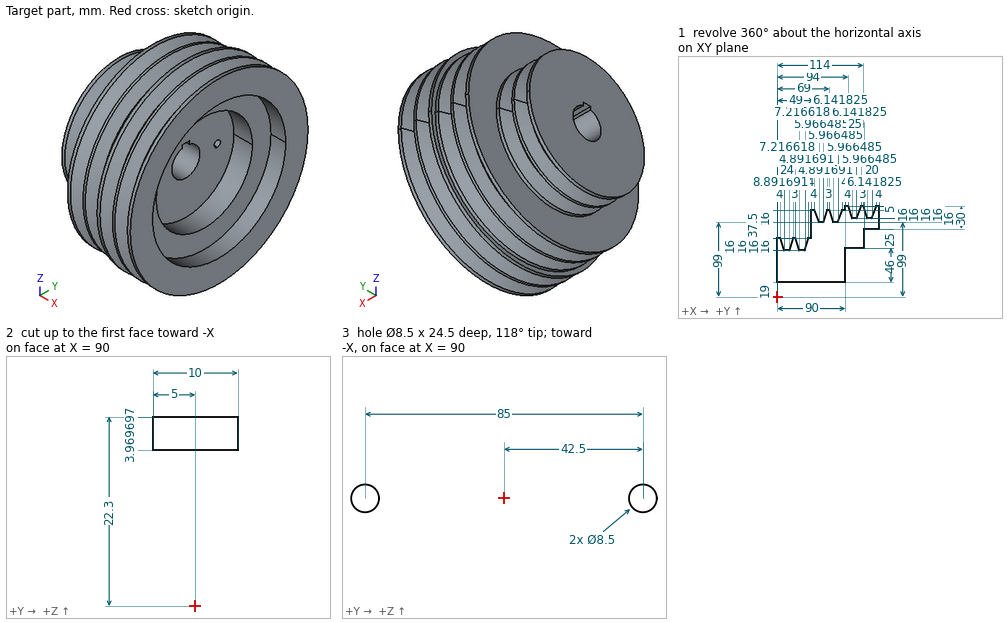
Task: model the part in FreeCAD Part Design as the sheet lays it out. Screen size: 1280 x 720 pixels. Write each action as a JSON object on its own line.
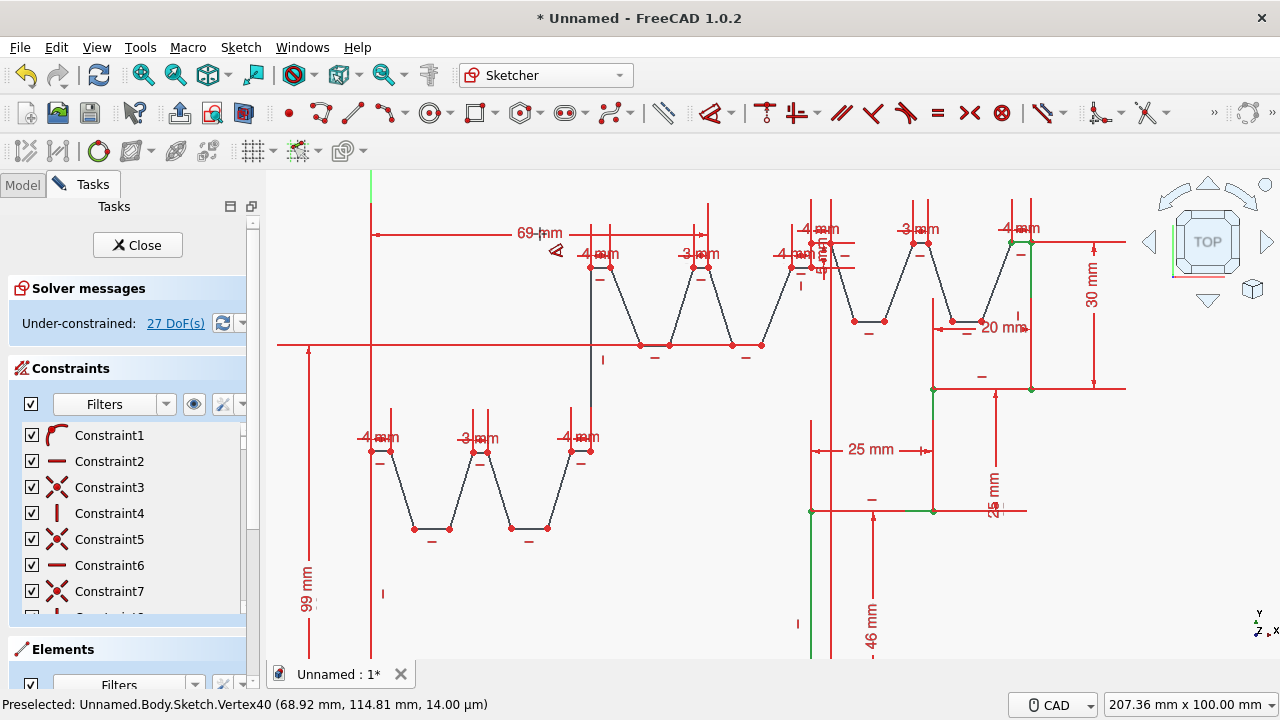
{"action": "left_click", "coordinate": [670, 346]}
{"action": "left_click", "coordinate": [337, 488]}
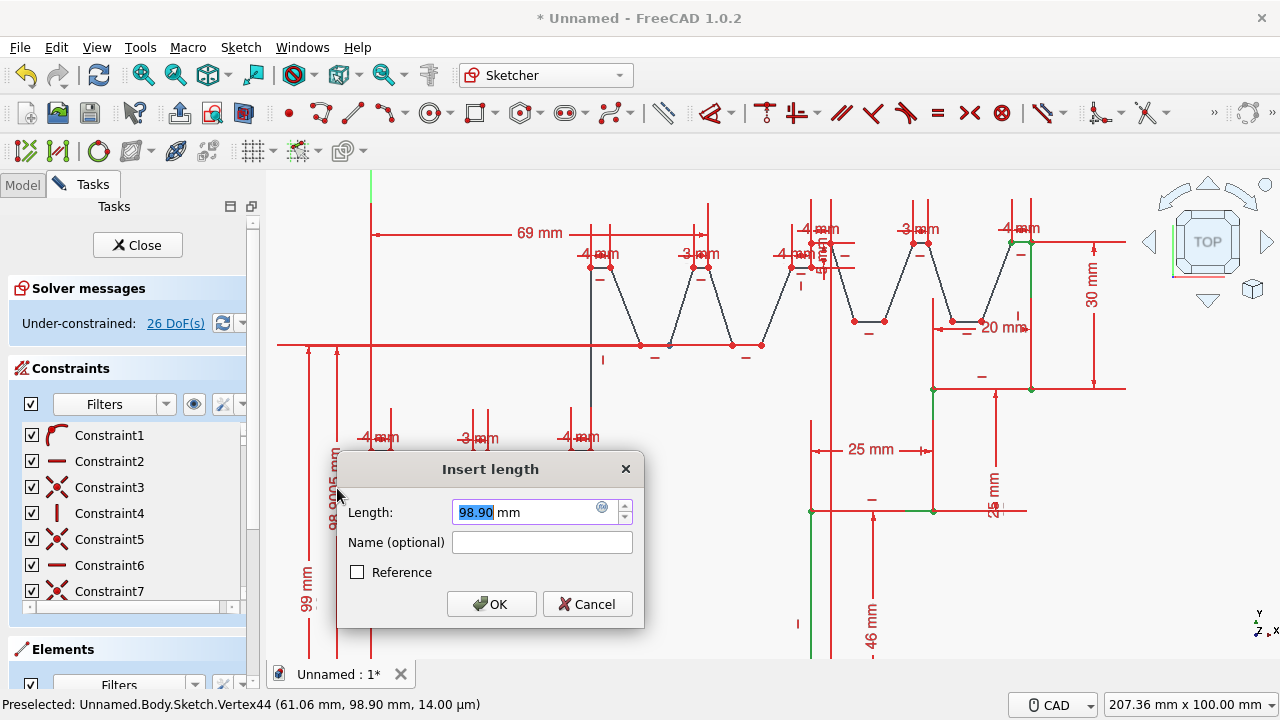
{"action": "type", "text": "99"}
{"action": "key", "text": "Return"}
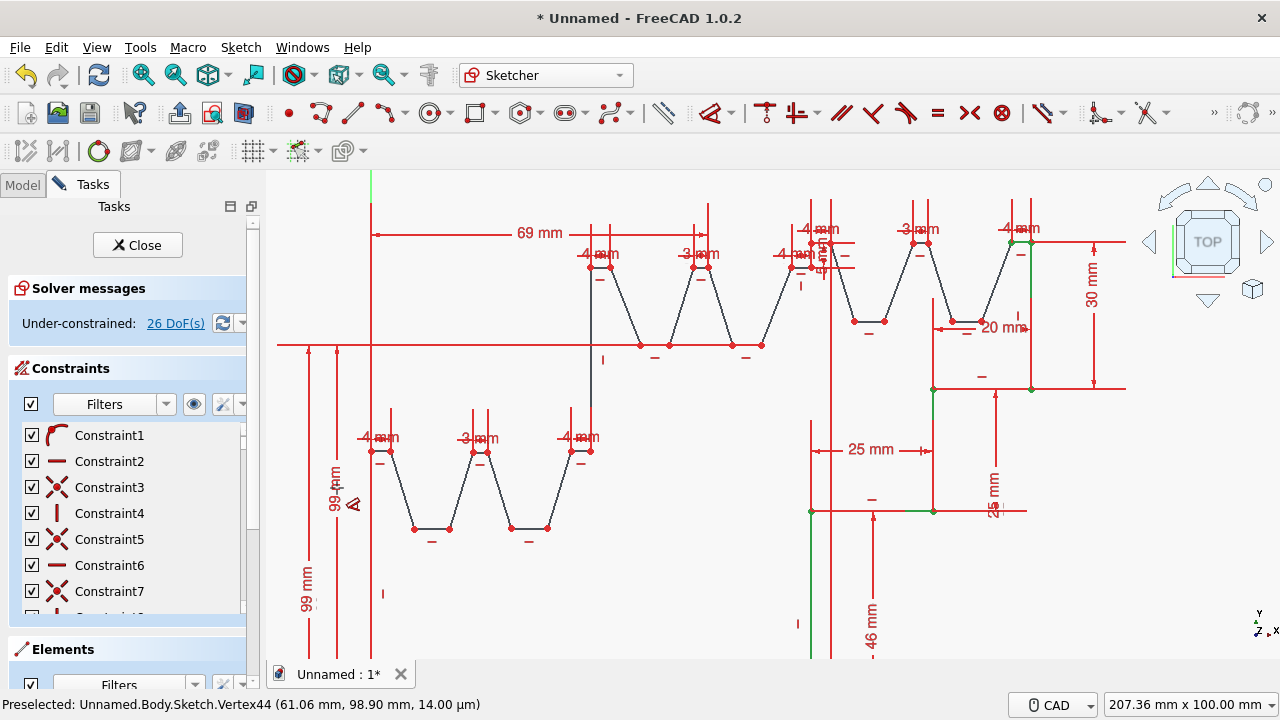
{"action": "left_click", "coordinate": [610, 268]}
{"action": "left_click", "coordinate": [436, 234]}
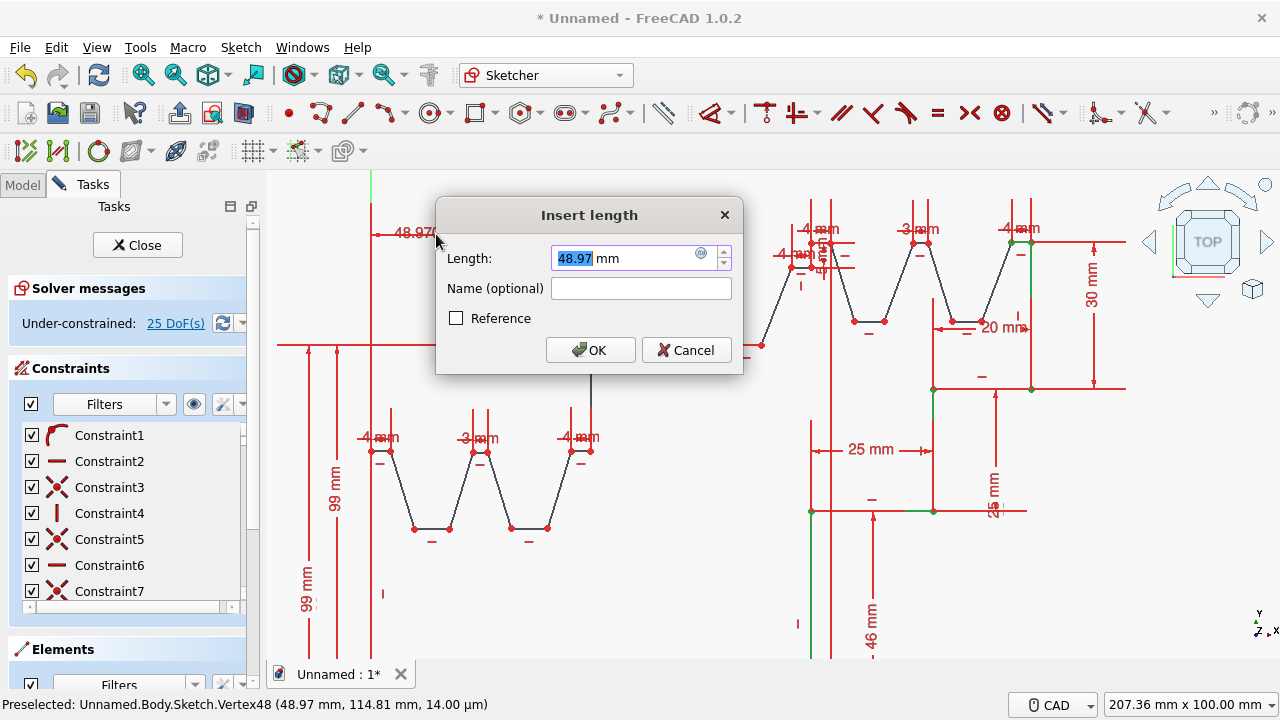
{"action": "type", "text": "49"}
{"action": "key", "text": "Return"}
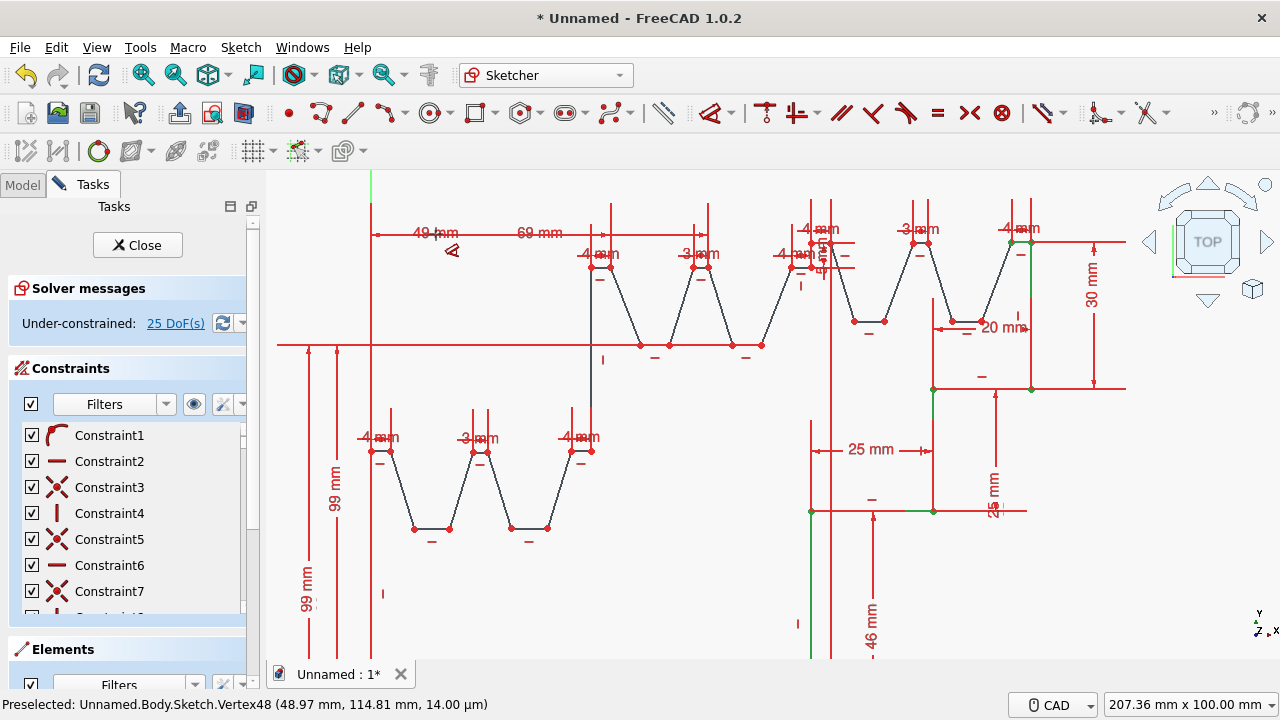
{"action": "left_click", "coordinate": [488, 453]}
{"action": "left_click", "coordinate": [429, 419]}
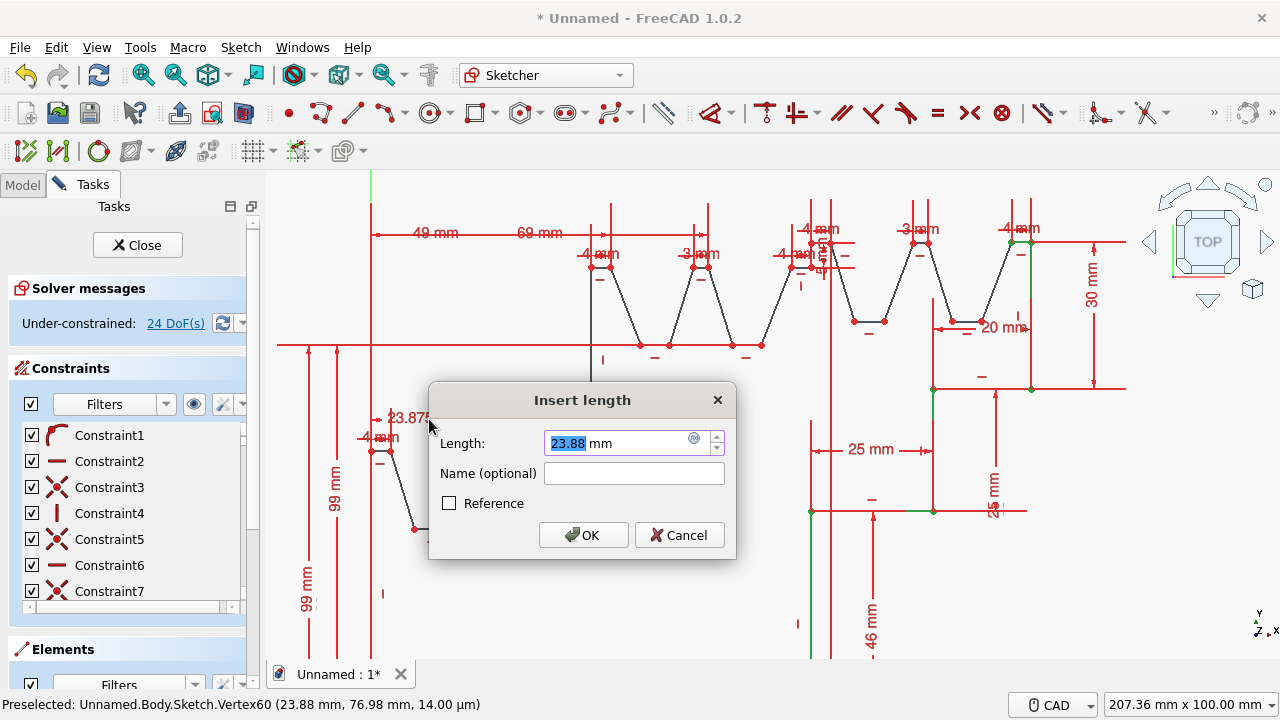
{"action": "type", "text": "24"}
{"action": "key", "text": "Return"}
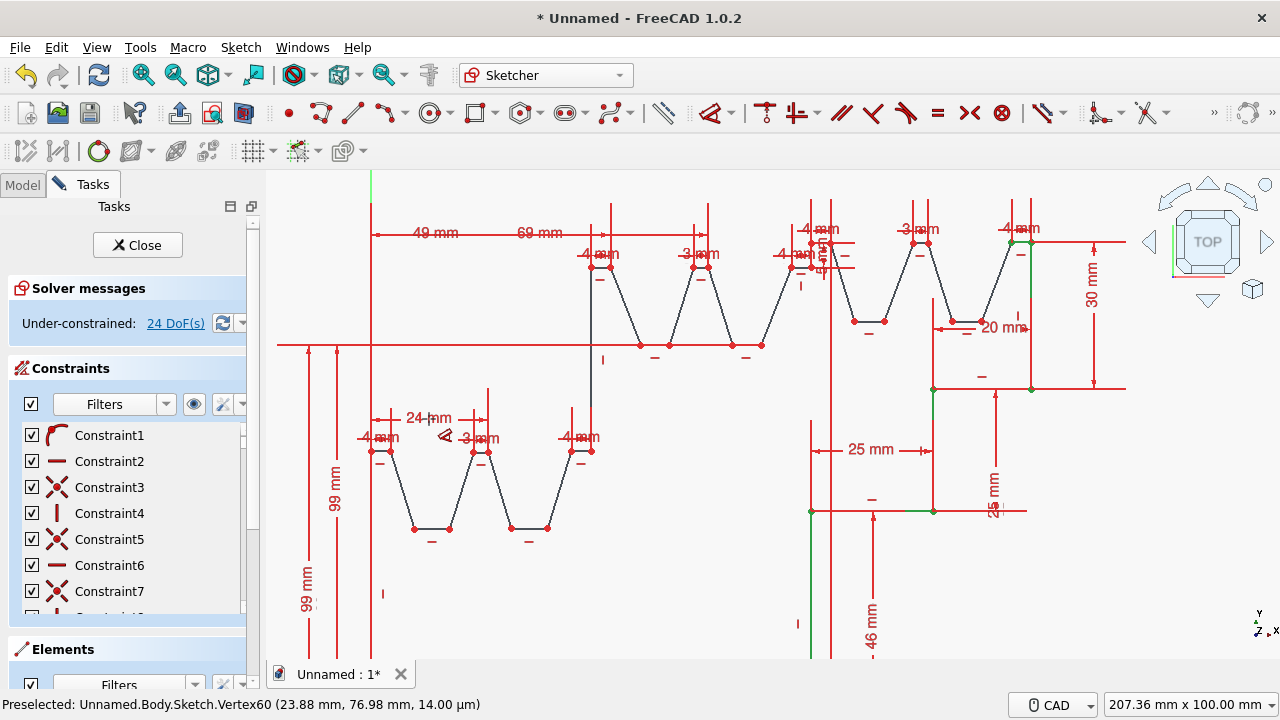
{"action": "left_click", "coordinate": [1003, 266]}
{"action": "left_click", "coordinate": [1046, 264]}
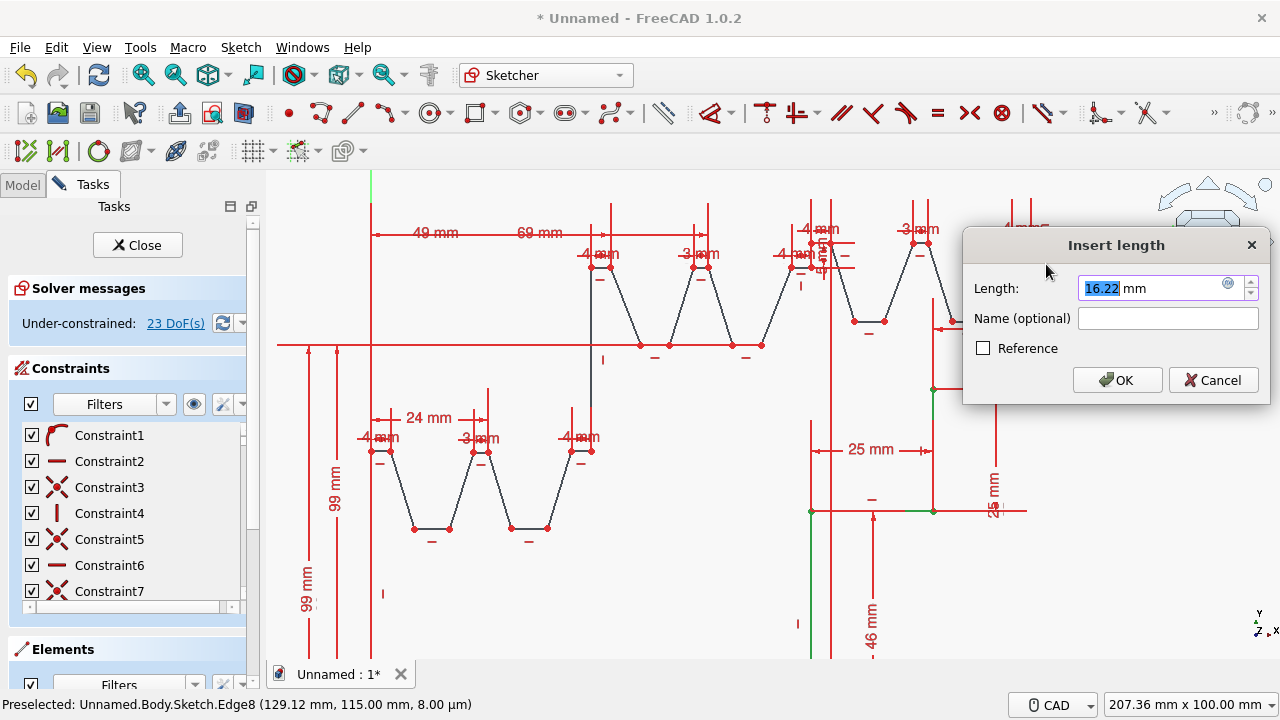
{"action": "type", "text": "16"}
{"action": "key", "text": "Return"}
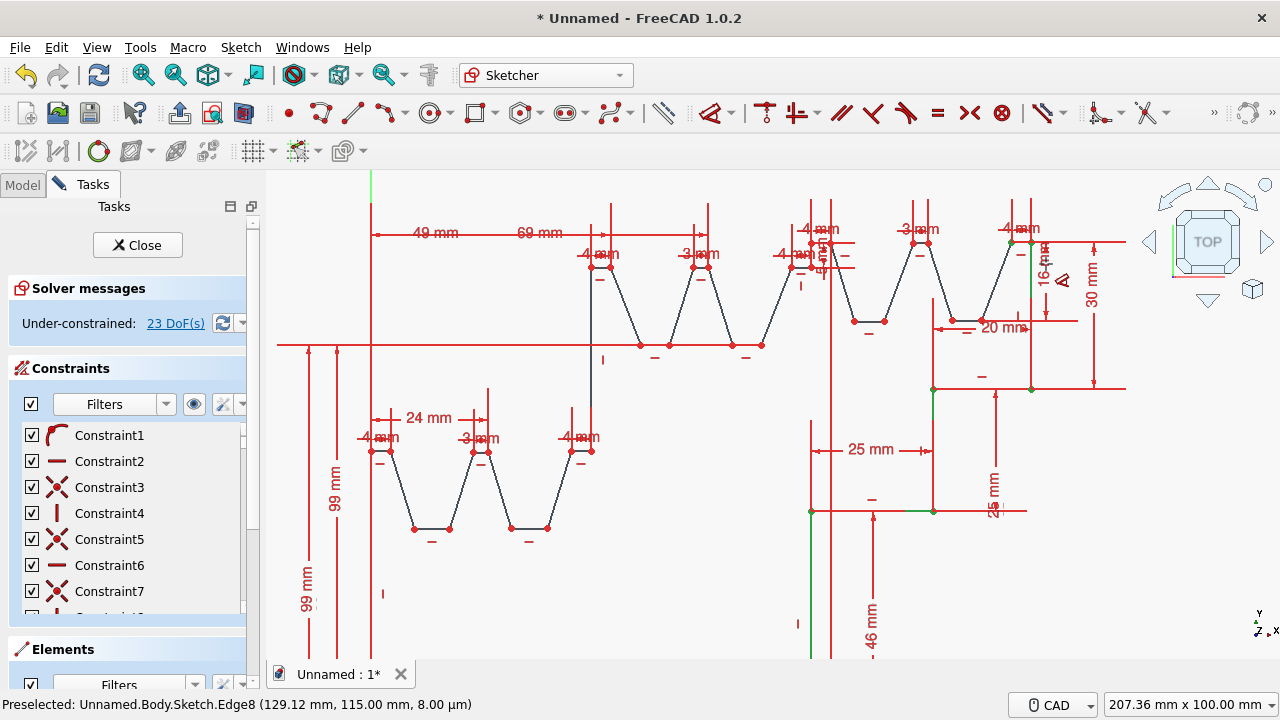
{"action": "left_click", "coordinate": [945, 297]}
{"action": "left_click", "coordinate": [894, 255]}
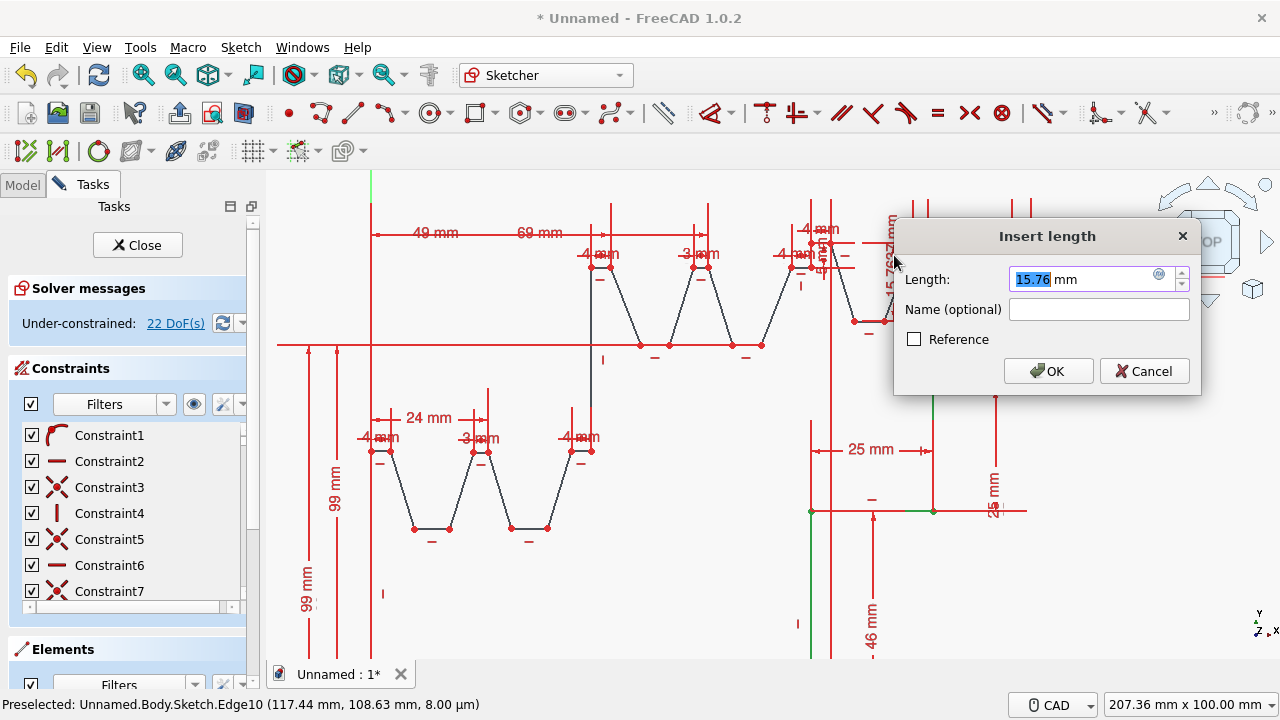
{"action": "type", "text": "16"}
{"action": "key", "text": "Return"}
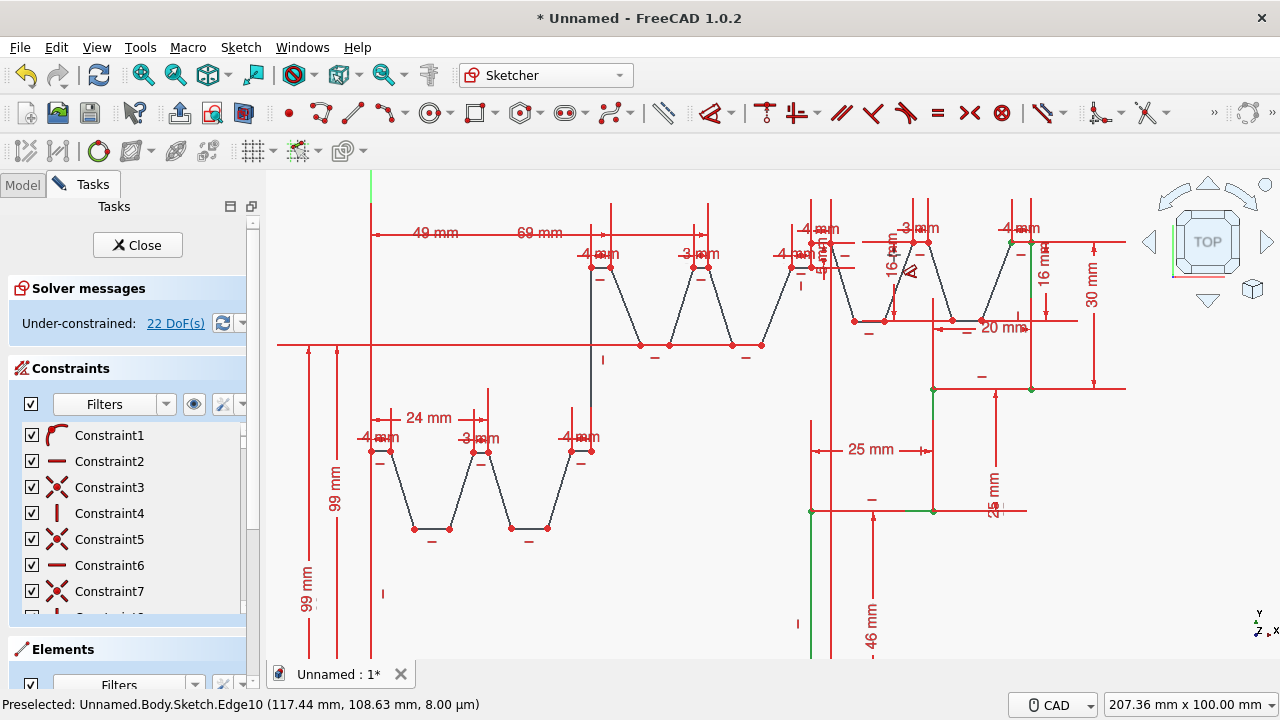
{"action": "left_click", "coordinate": [905, 266]}
{"action": "left_click", "coordinate": [971, 282]}